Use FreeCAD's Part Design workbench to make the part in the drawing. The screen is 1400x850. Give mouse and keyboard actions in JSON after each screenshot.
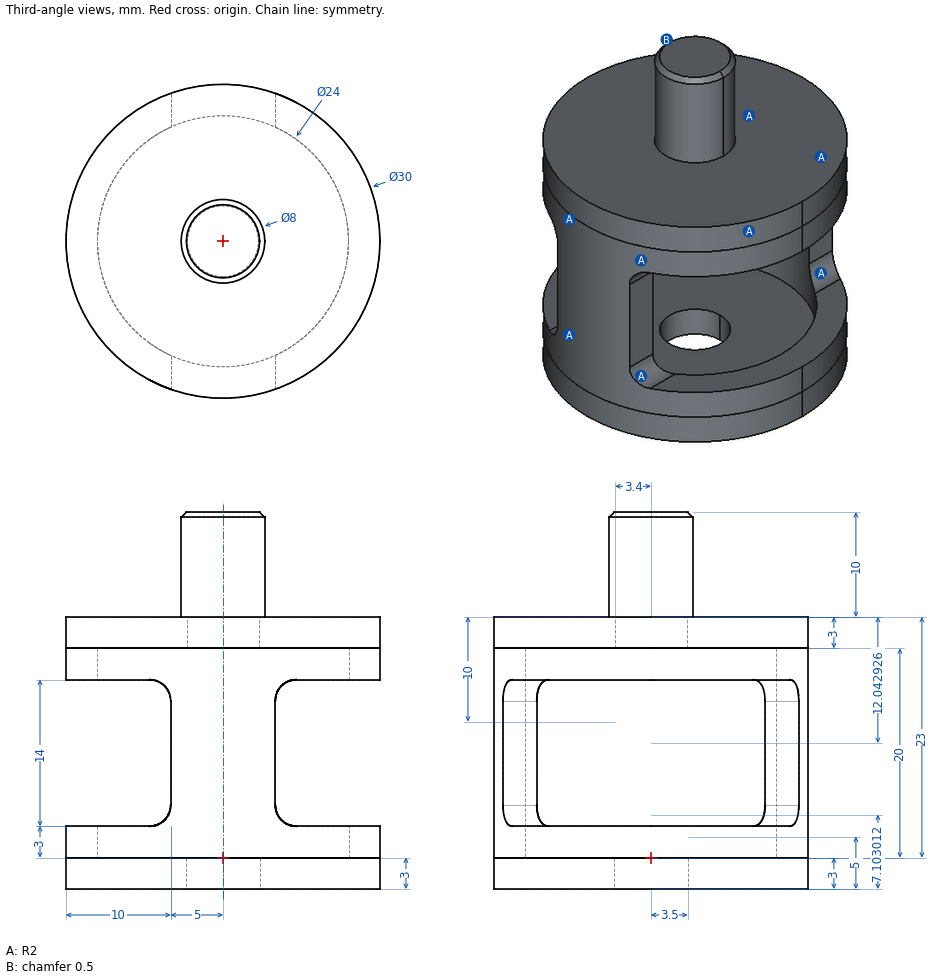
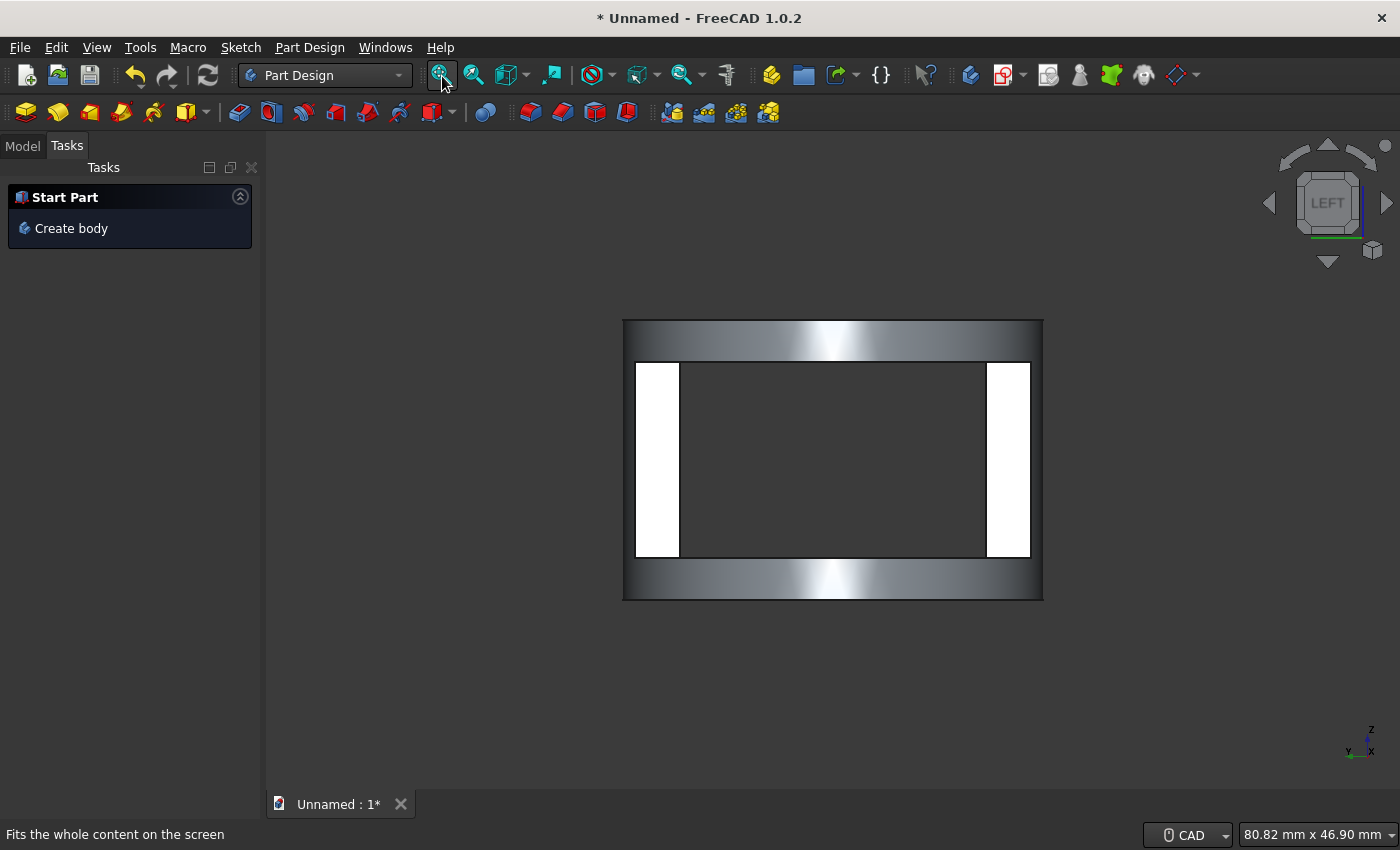
{"action": "left_click", "coordinate": [442, 76]}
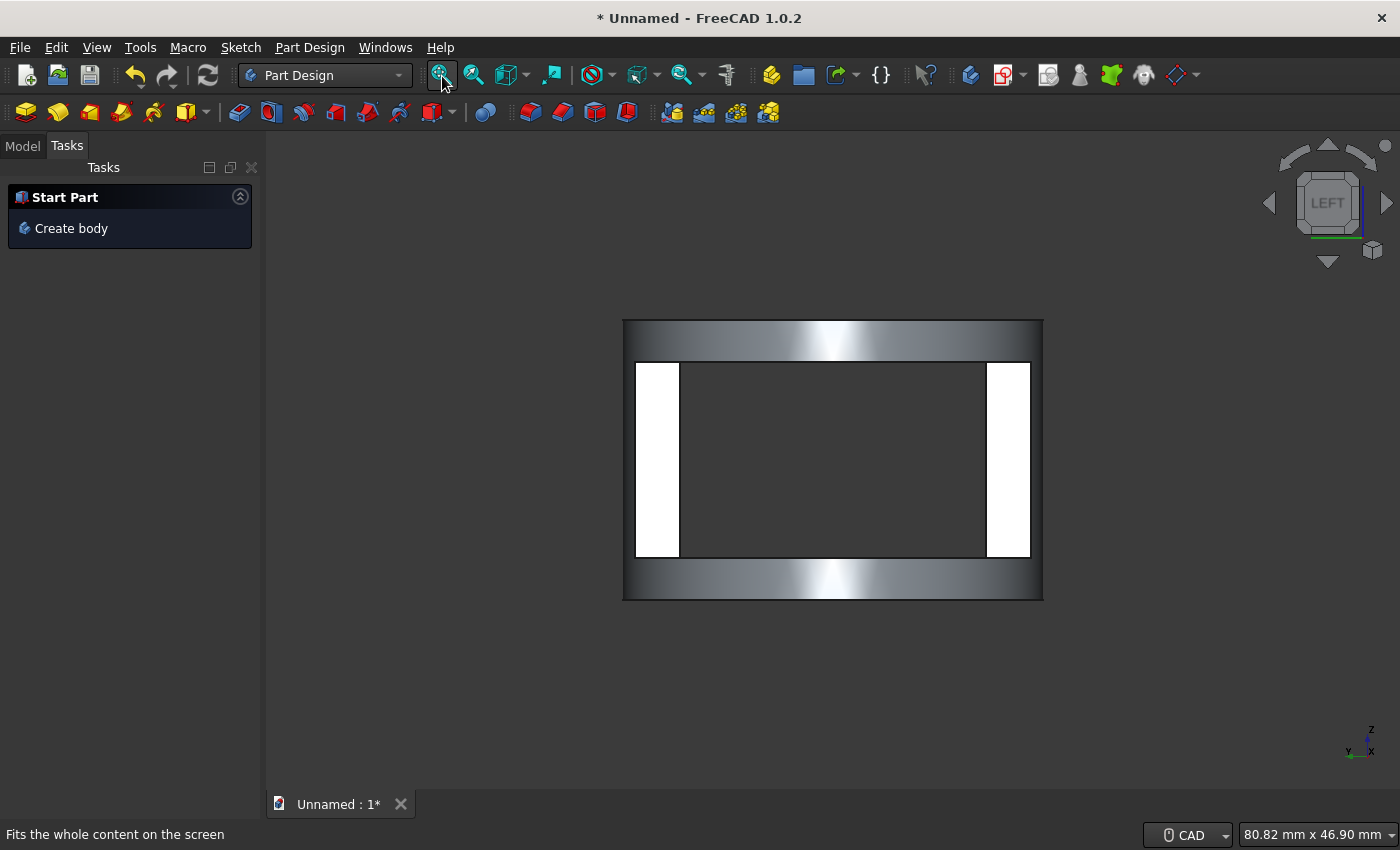
{"action": "key", "text": "v 3"}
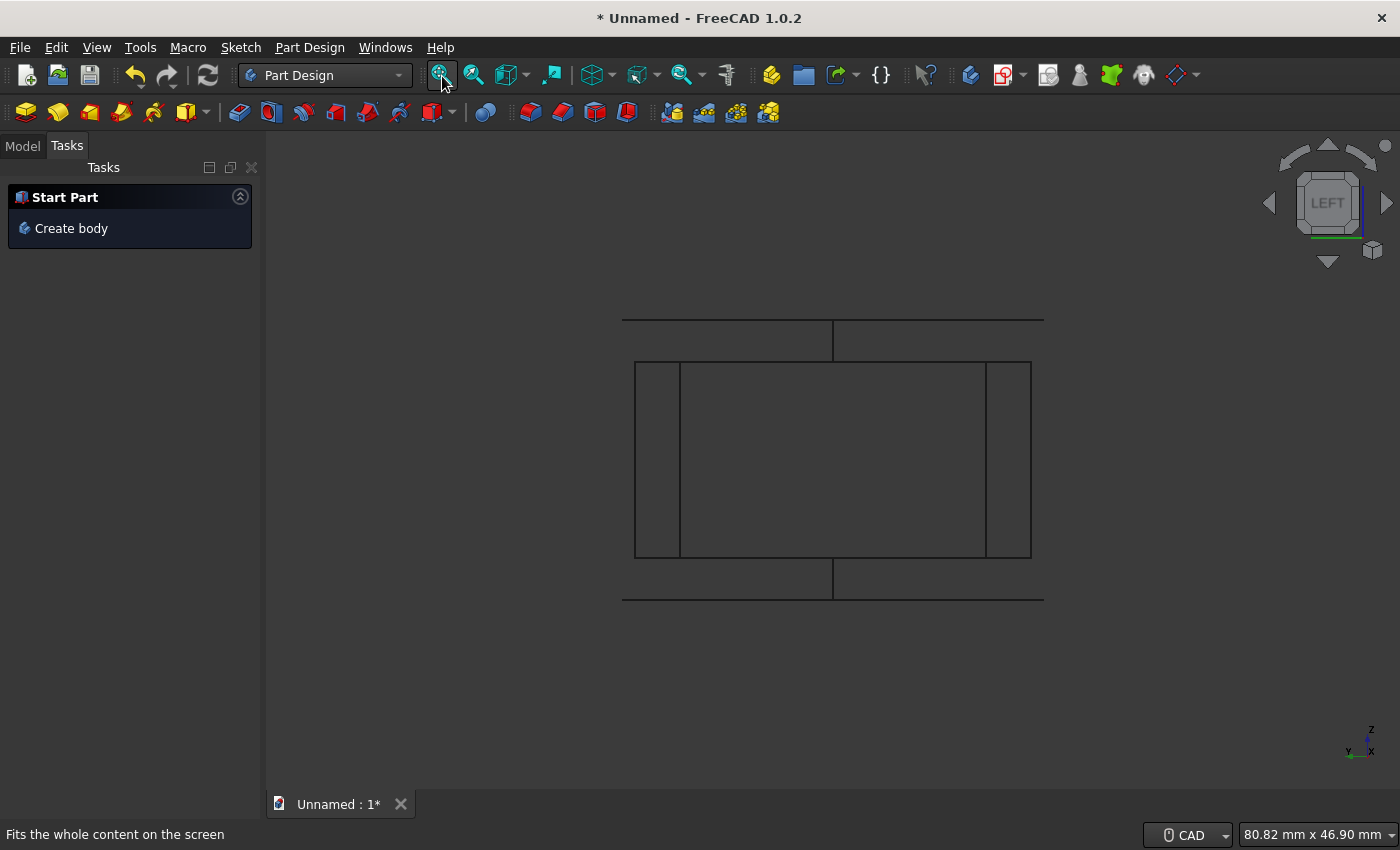
{"action": "key", "text": "0"}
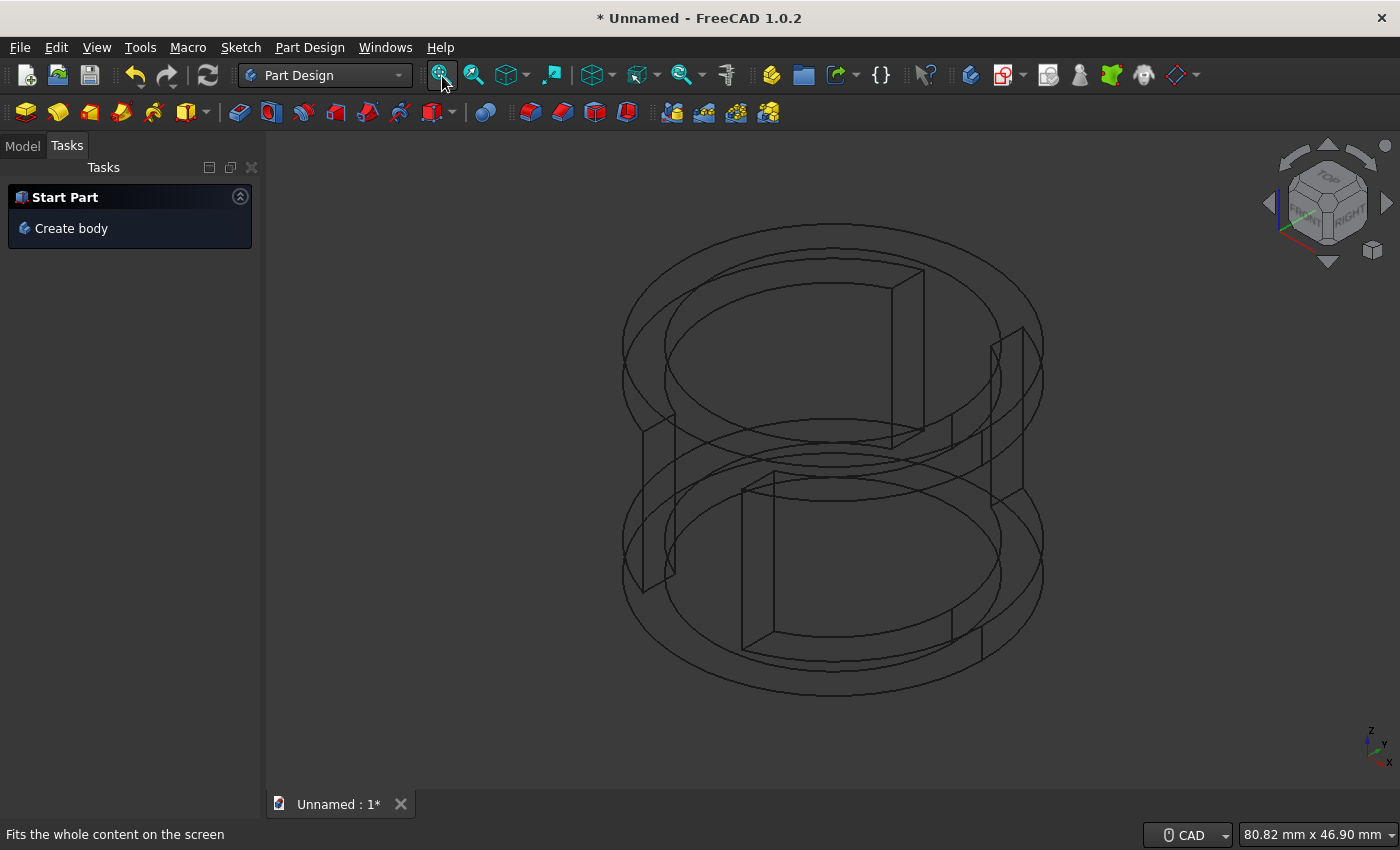
{"action": "left_click", "coordinate": [659, 582]}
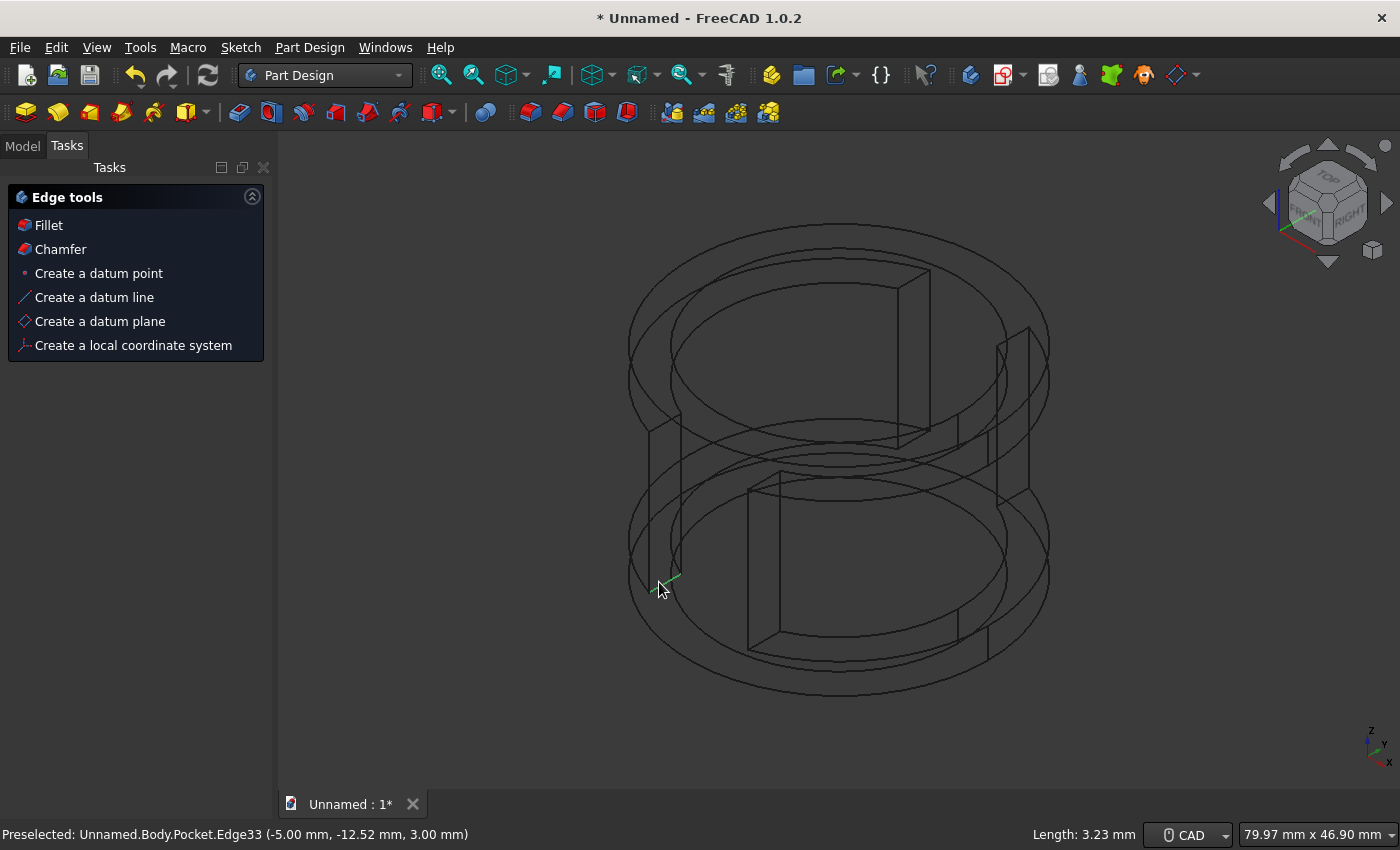
{"action": "left_click", "coordinate": [914, 439], "text": "ctrl"}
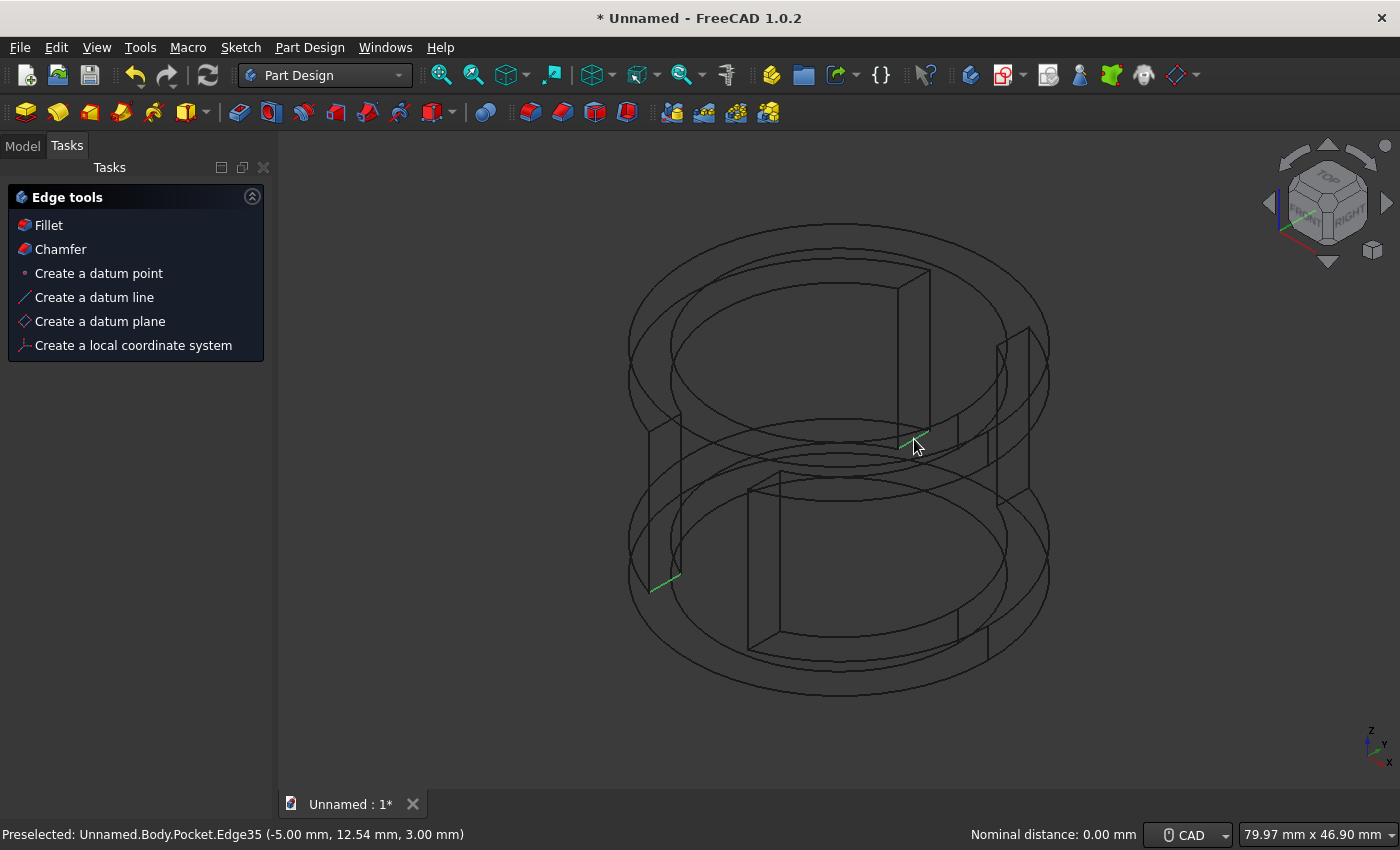
{"action": "left_click", "coordinate": [914, 278], "text": "ctrl"}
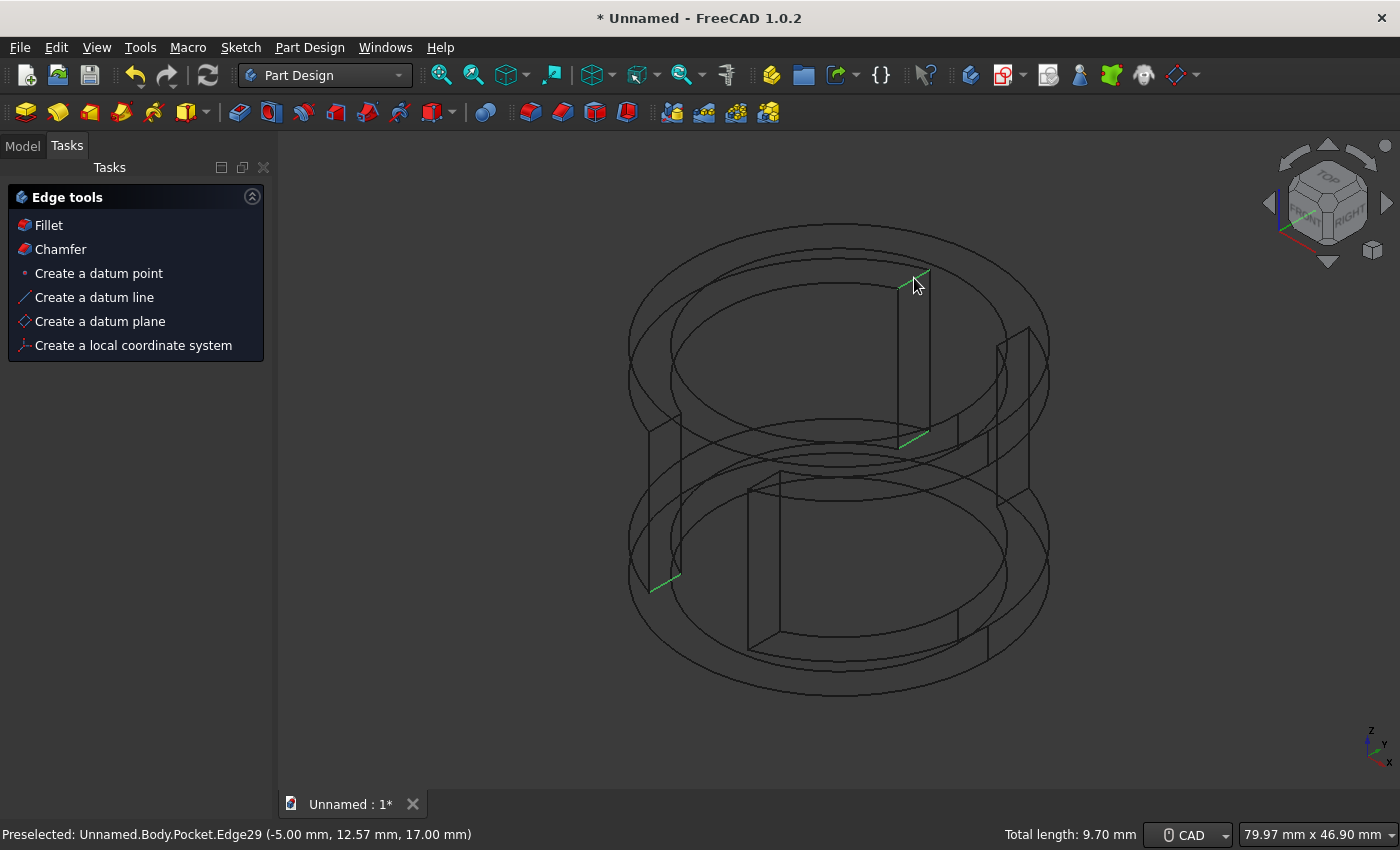
{"action": "left_click", "coordinate": [665, 422], "text": "ctrl"}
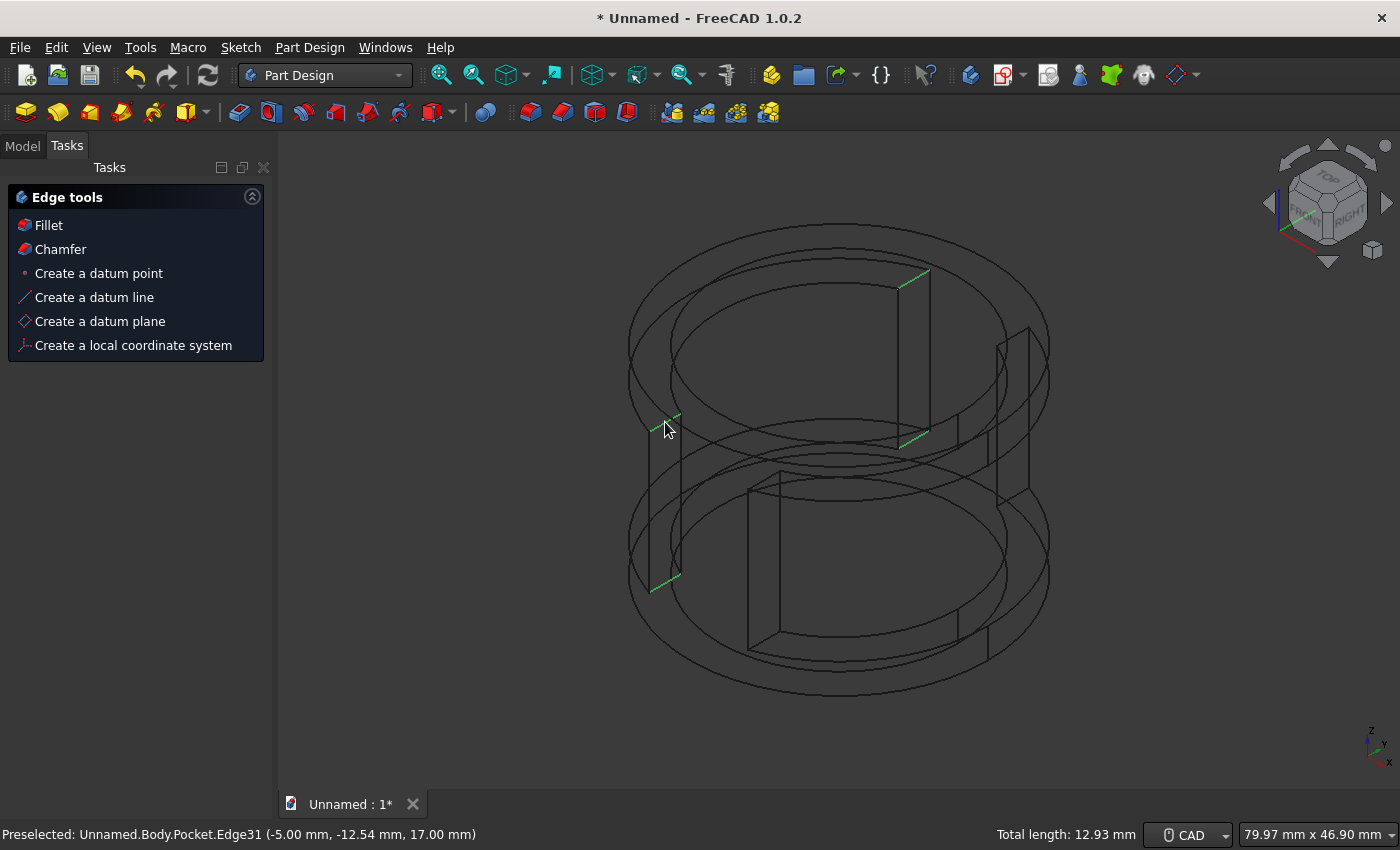
{"action": "left_click", "coordinate": [1013, 496], "text": "ctrl"}